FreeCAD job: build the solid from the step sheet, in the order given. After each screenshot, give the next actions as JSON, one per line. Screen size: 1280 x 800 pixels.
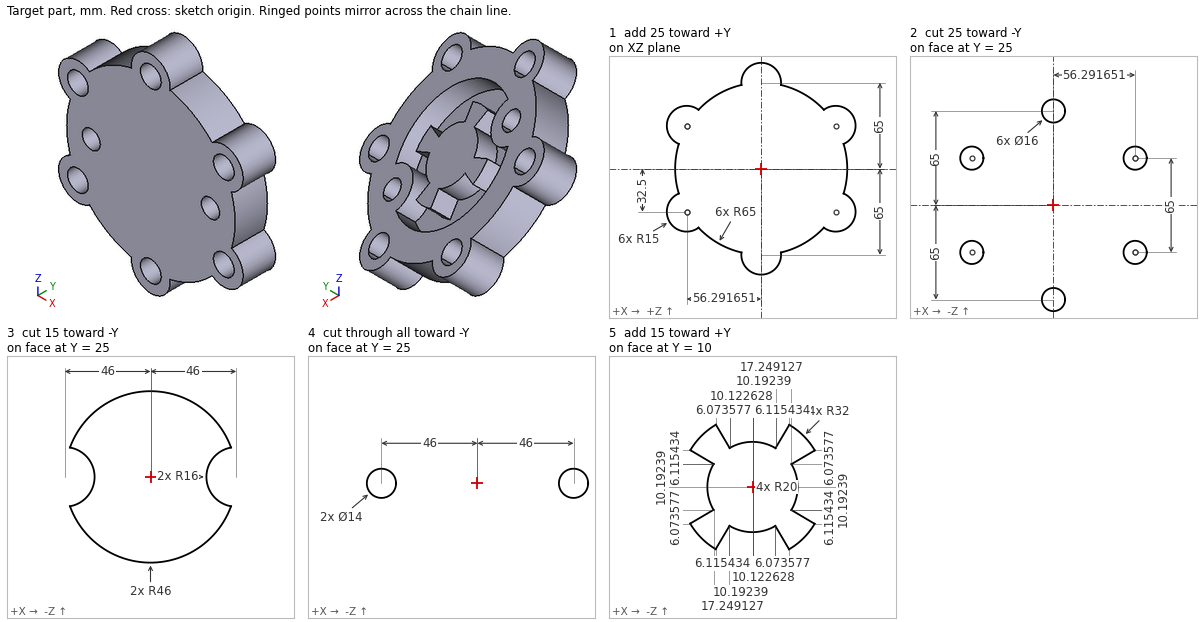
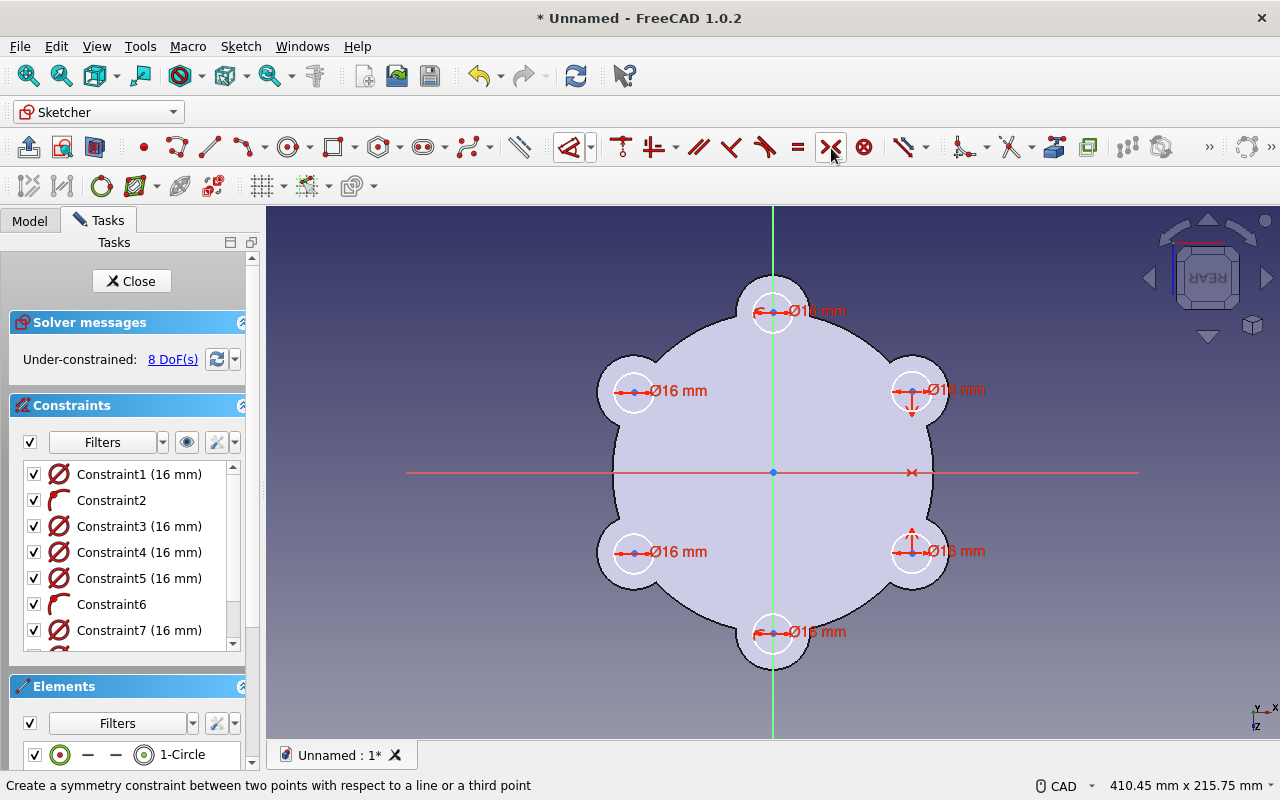
{"action": "left_click", "coordinate": [912, 553]}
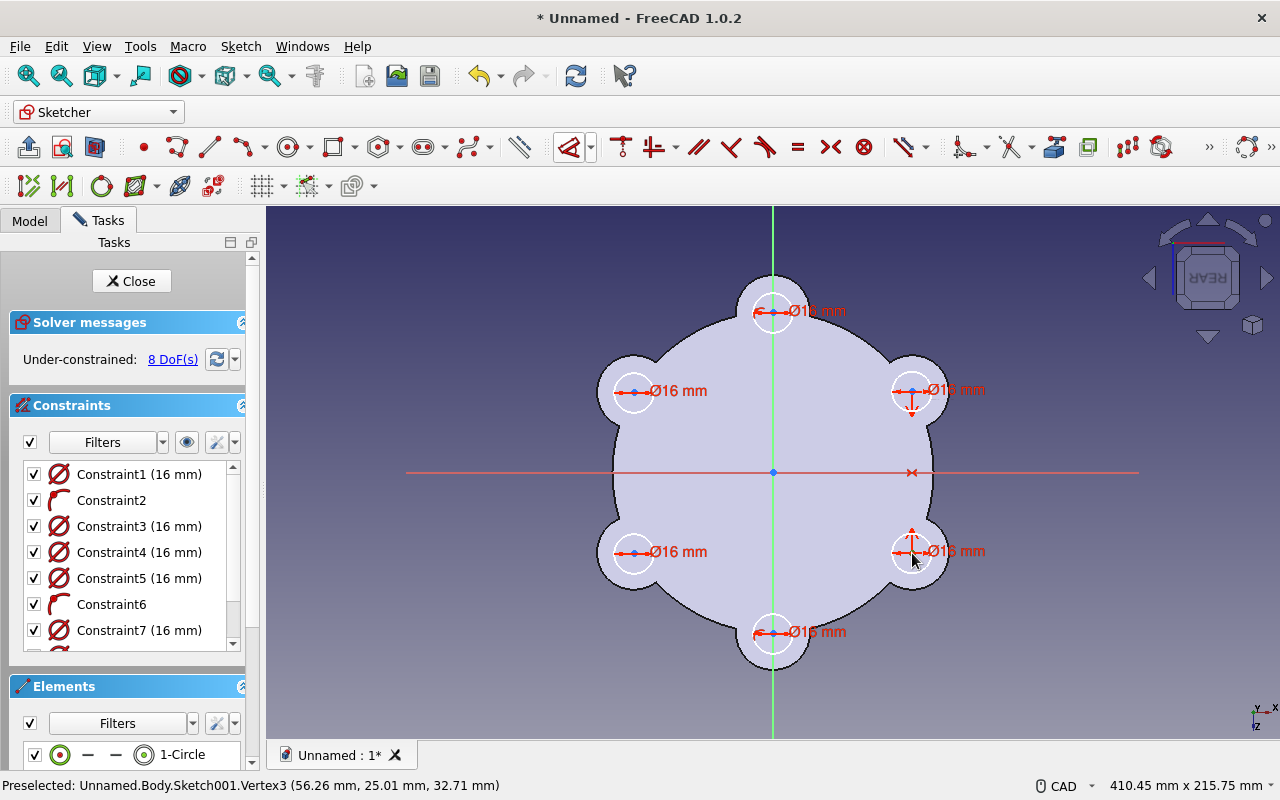
{"action": "left_click", "coordinate": [634, 554]}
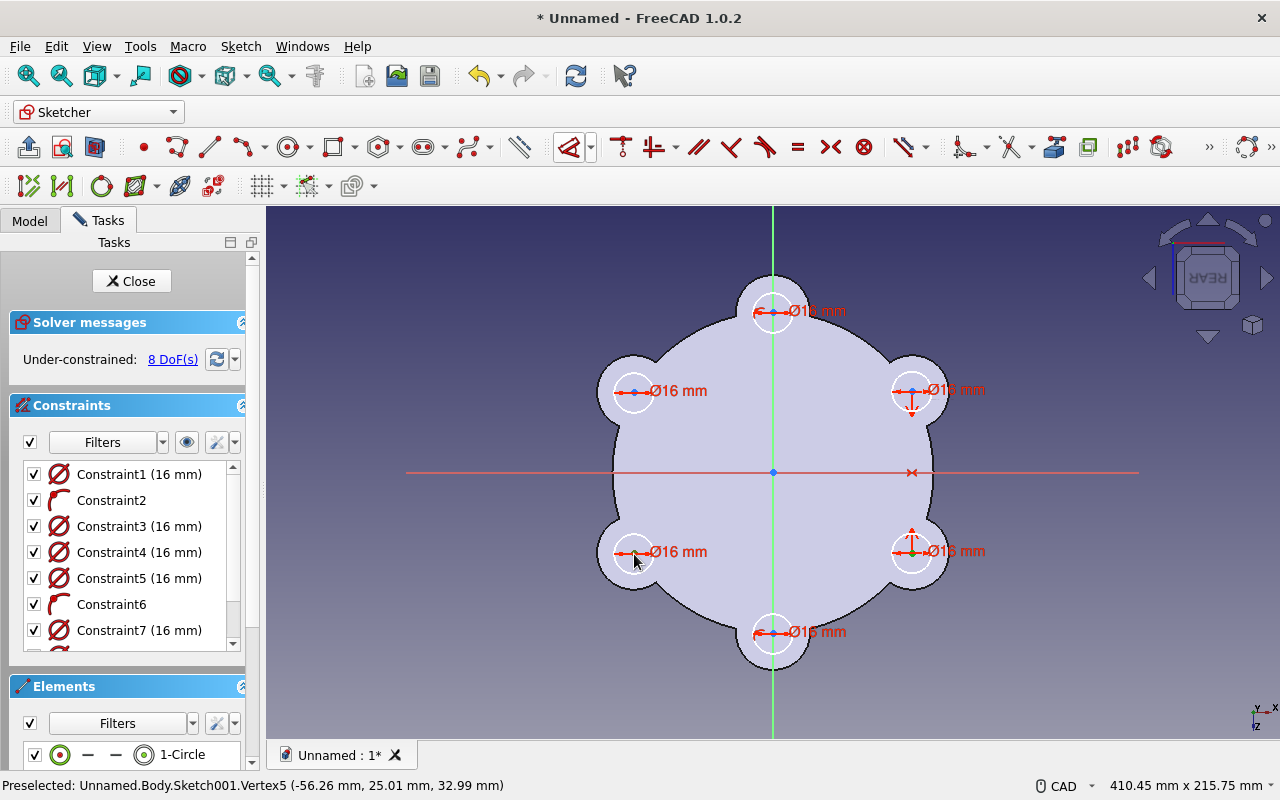
{"action": "left_click", "coordinate": [773, 575]}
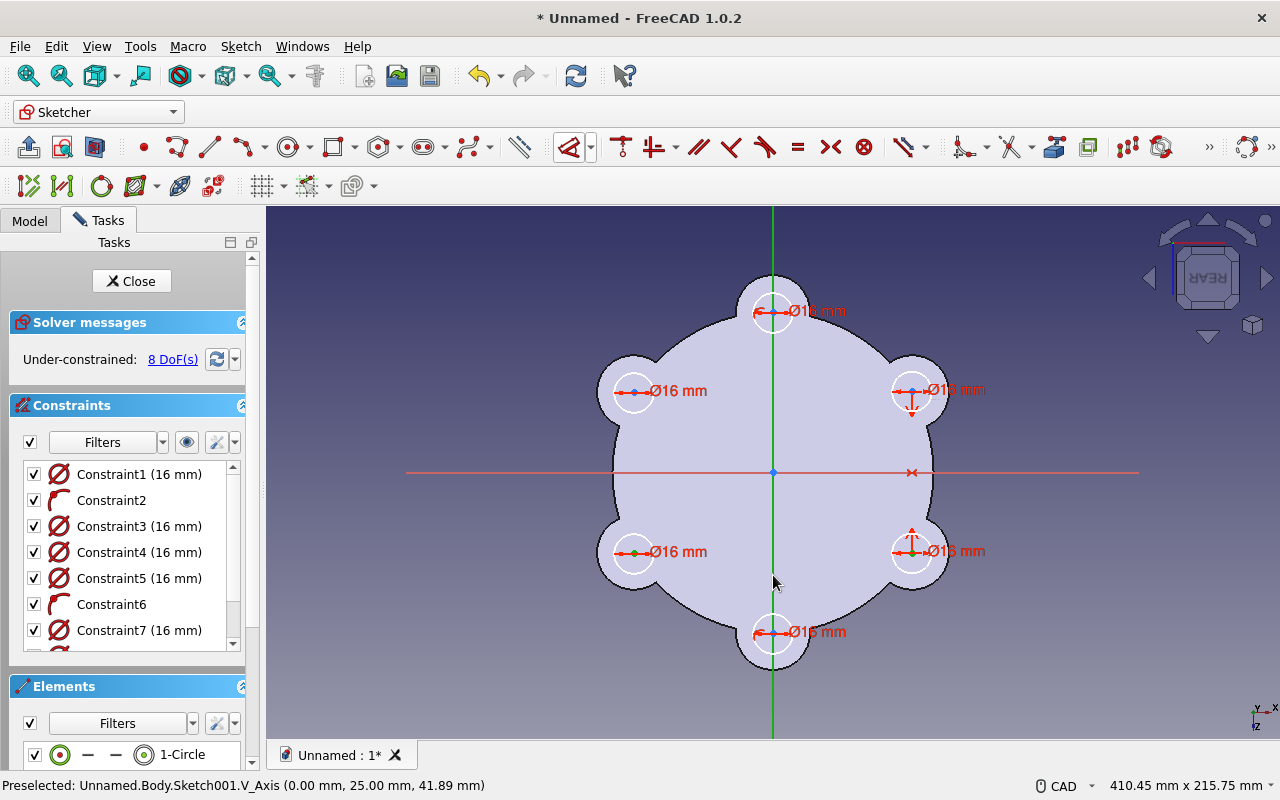
{"action": "key", "text": "s"}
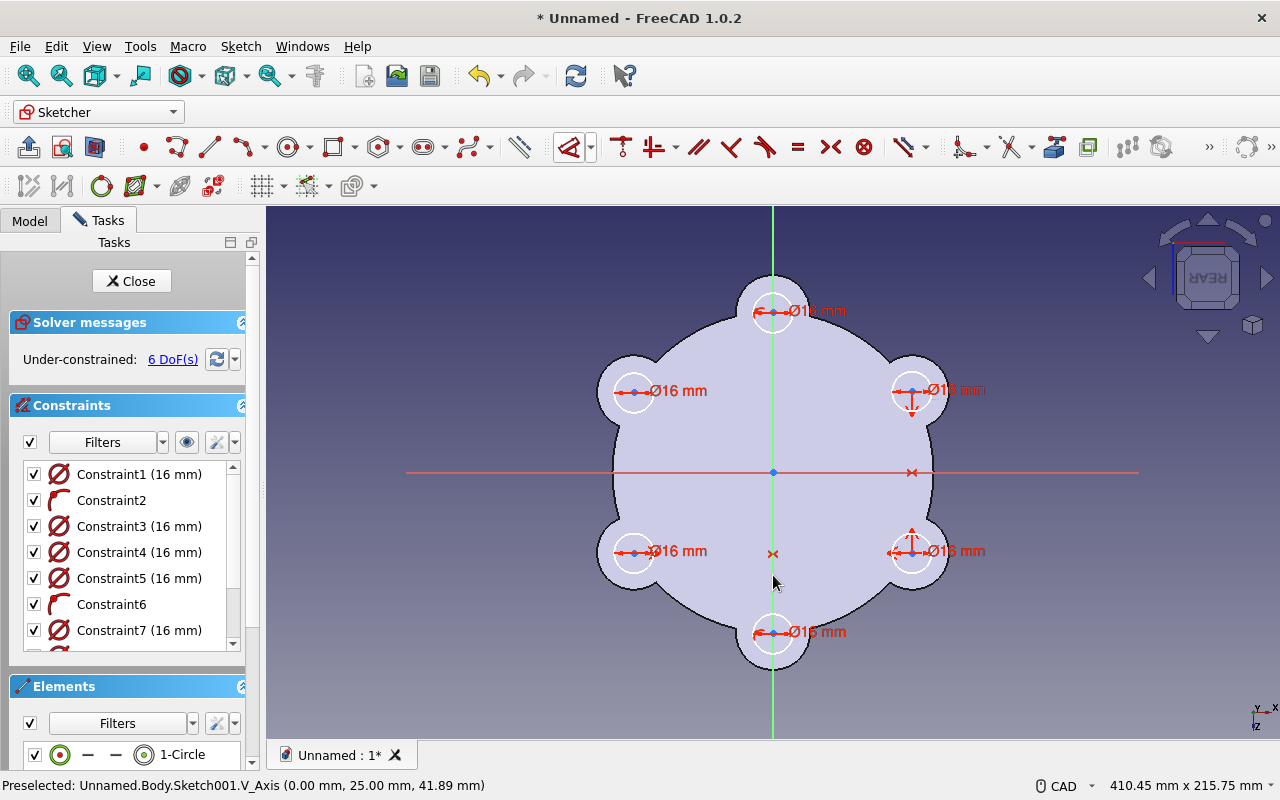
{"action": "left_click", "coordinate": [912, 392]}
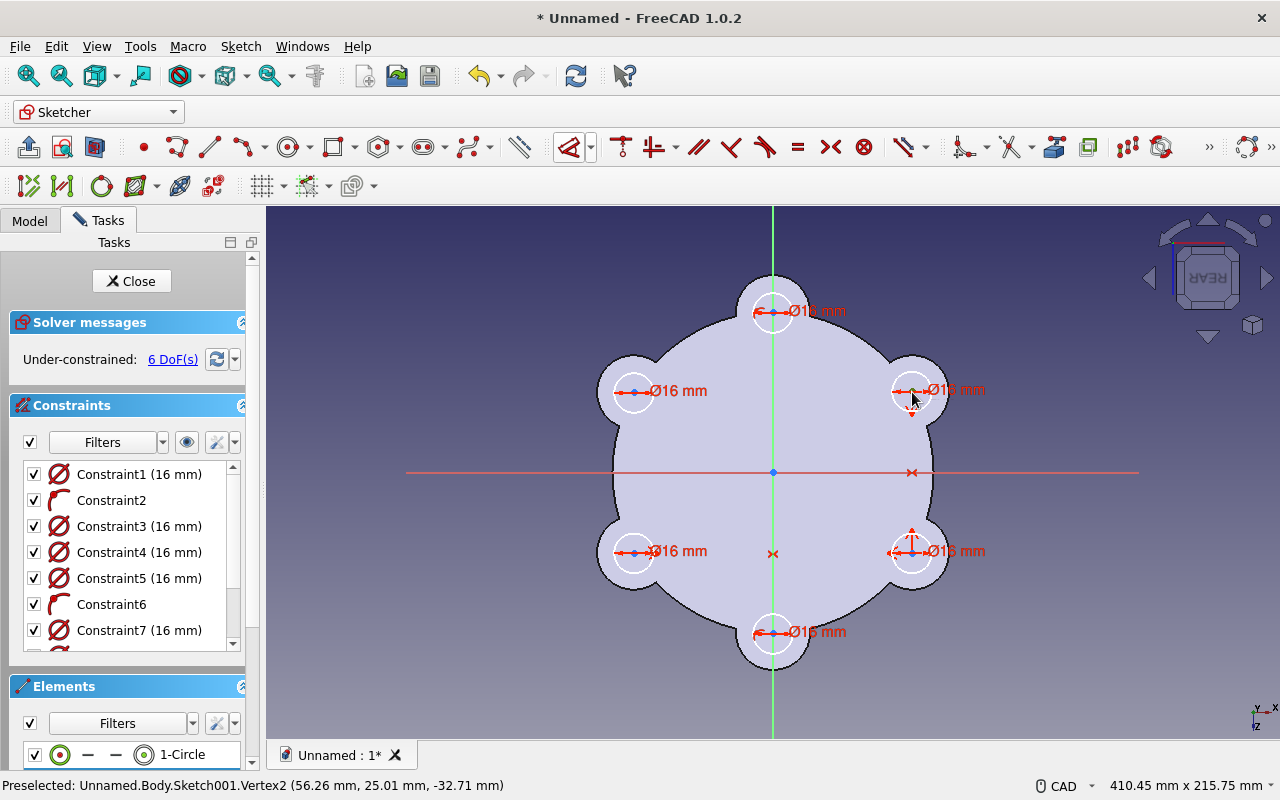
{"action": "left_click", "coordinate": [634, 393]}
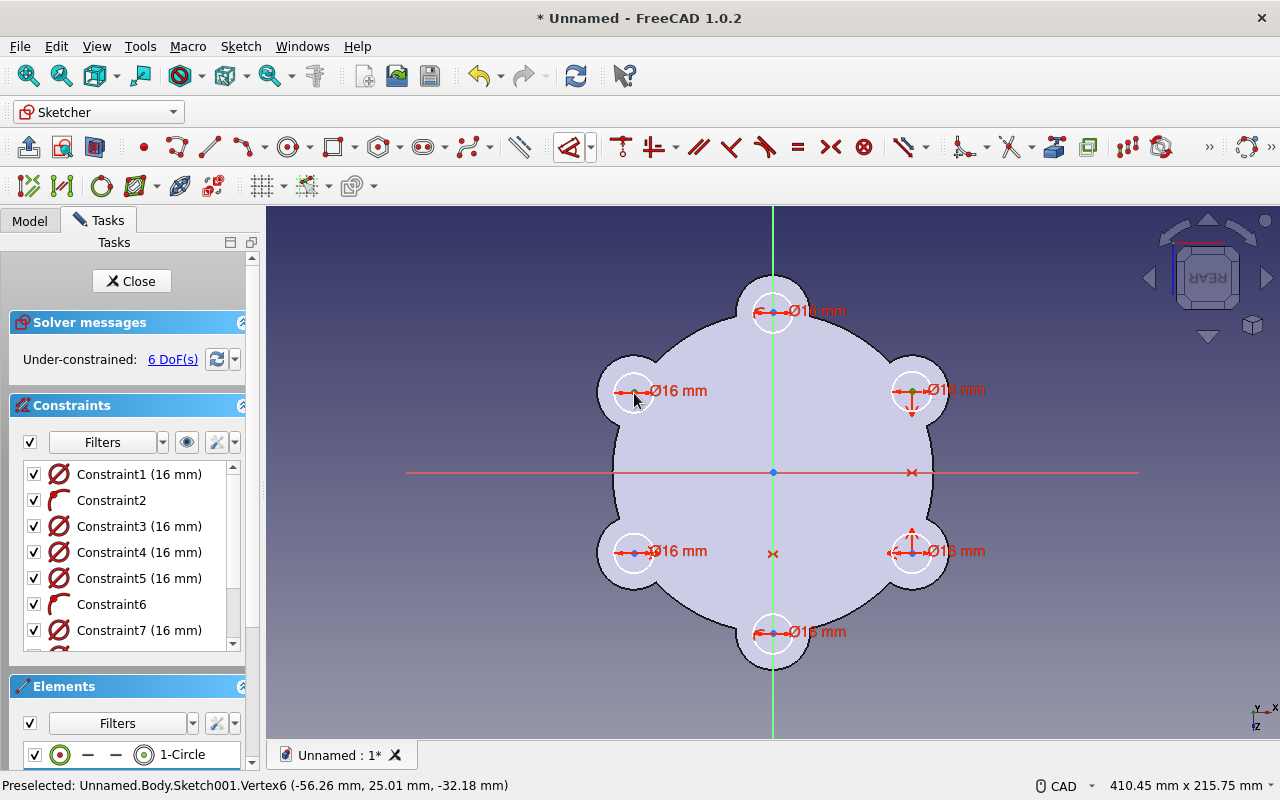
{"action": "left_click", "coordinate": [773, 575]}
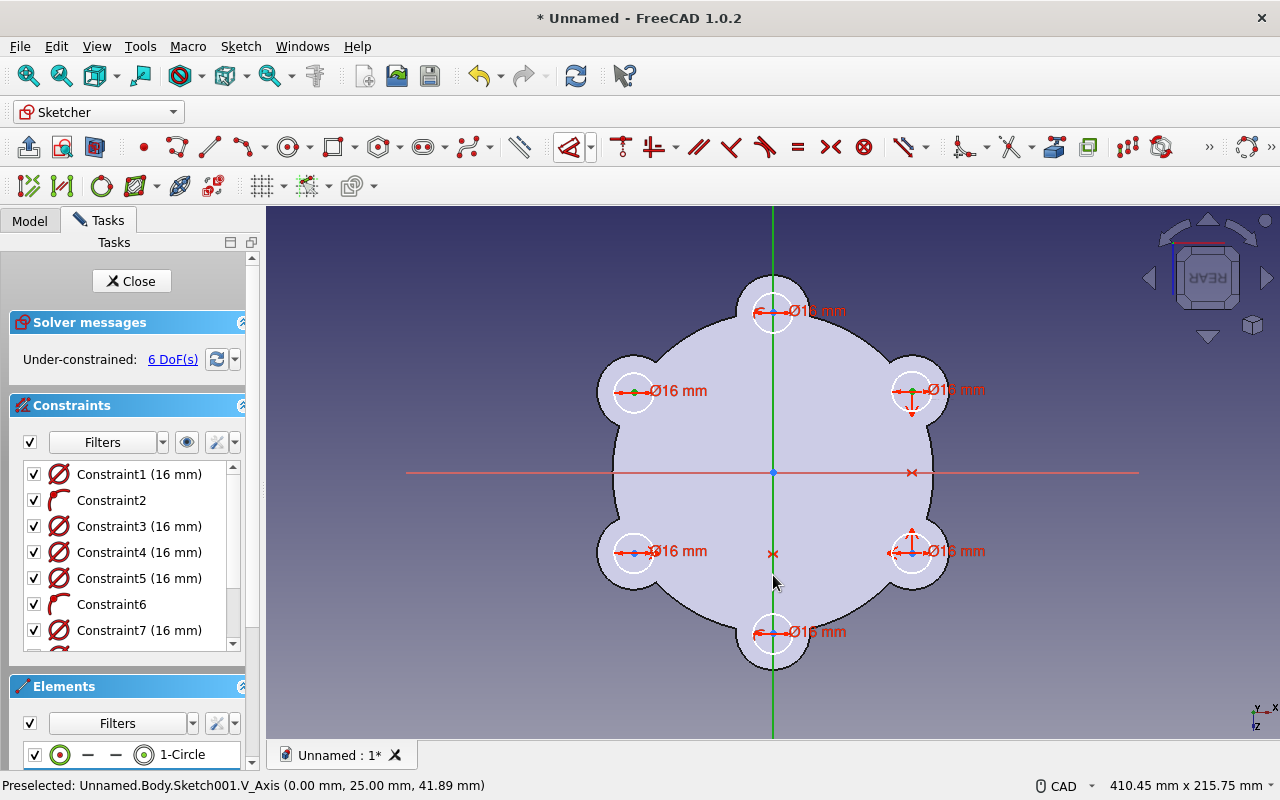
{"action": "key", "text": "s"}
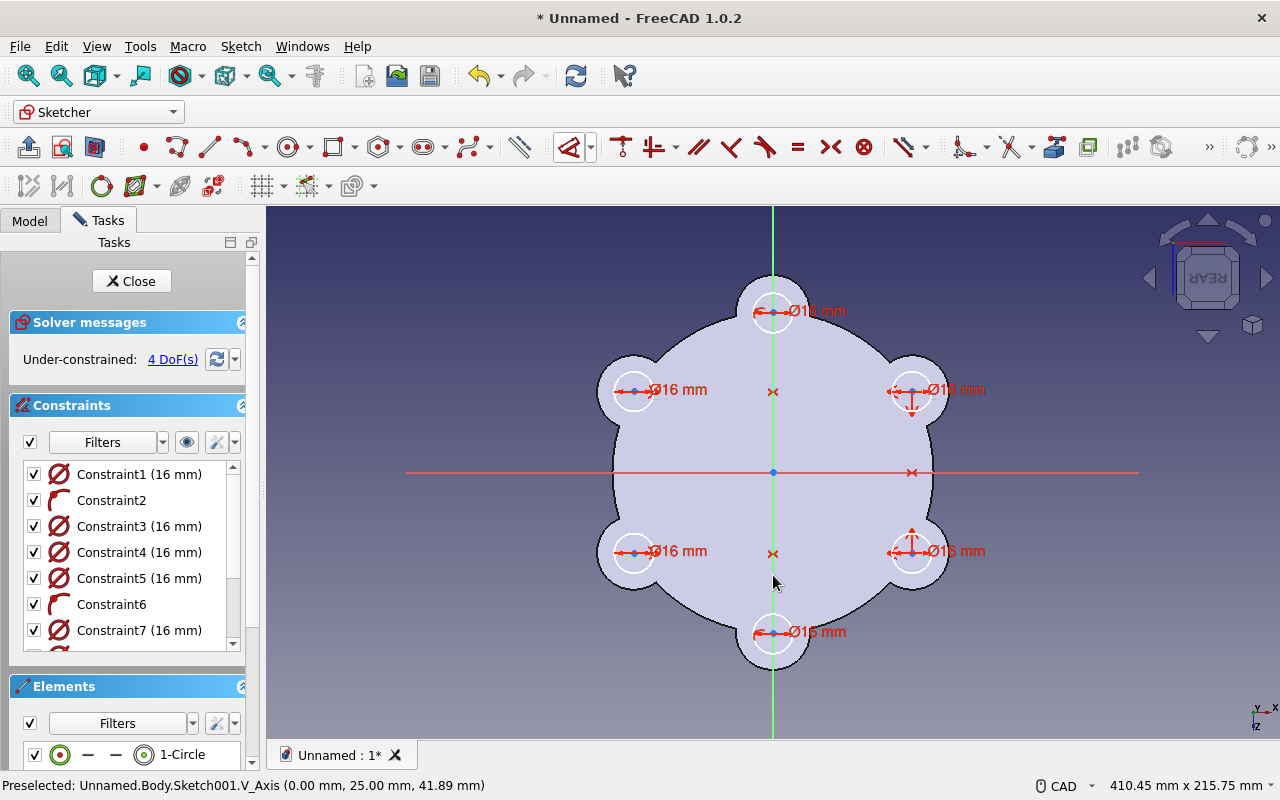
{"action": "left_click", "coordinate": [773, 313]}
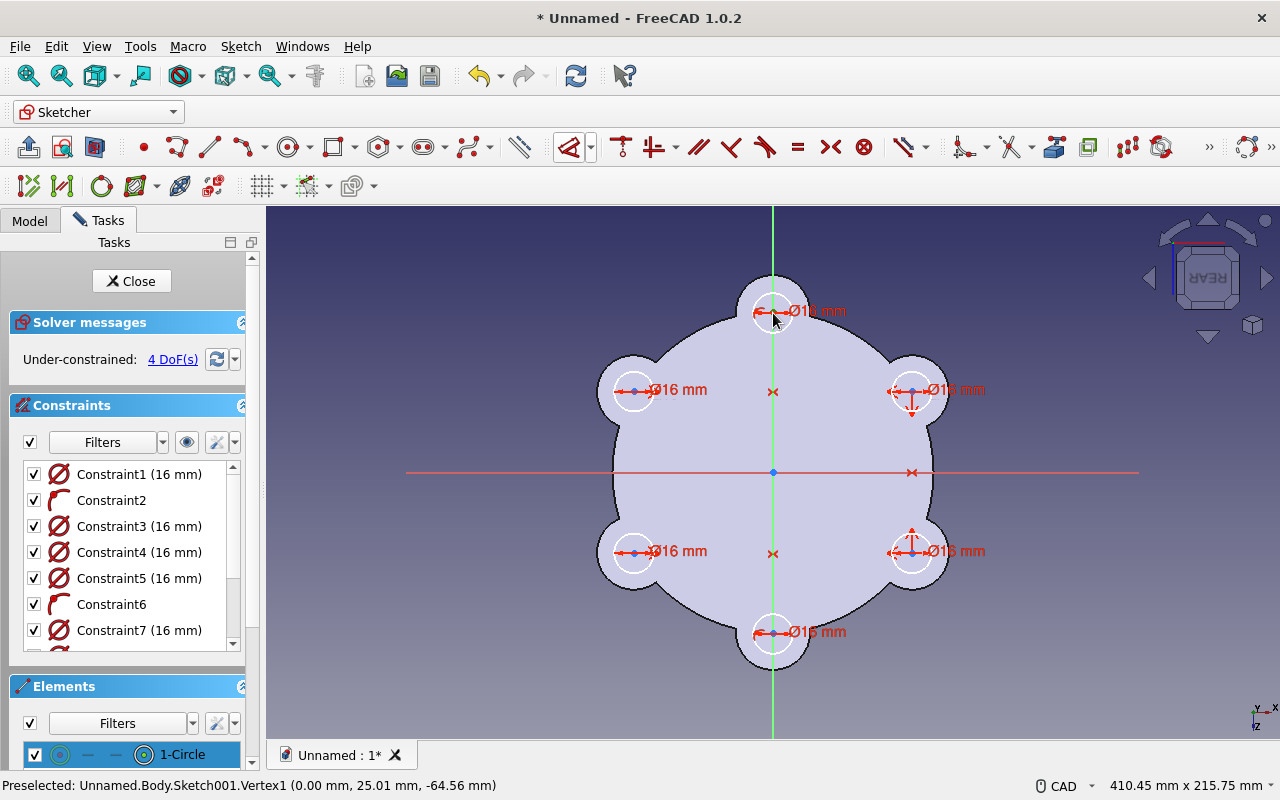
{"action": "key", "text": "i"}